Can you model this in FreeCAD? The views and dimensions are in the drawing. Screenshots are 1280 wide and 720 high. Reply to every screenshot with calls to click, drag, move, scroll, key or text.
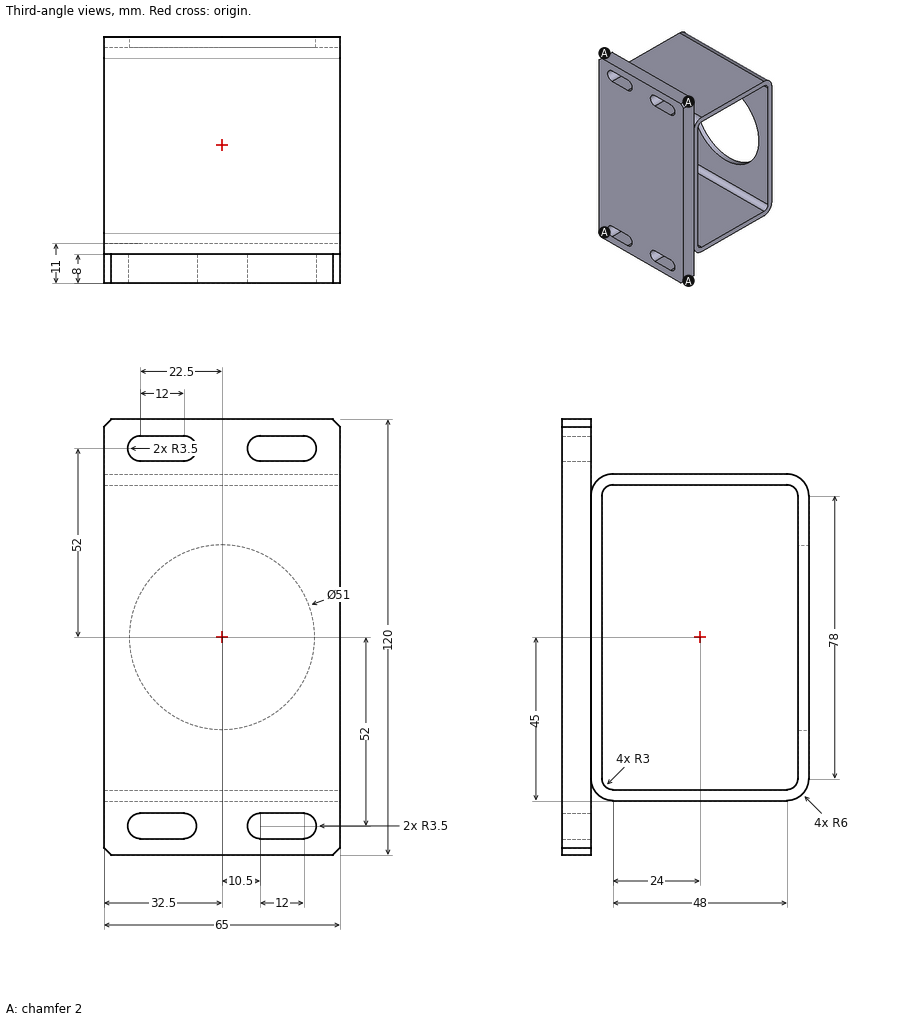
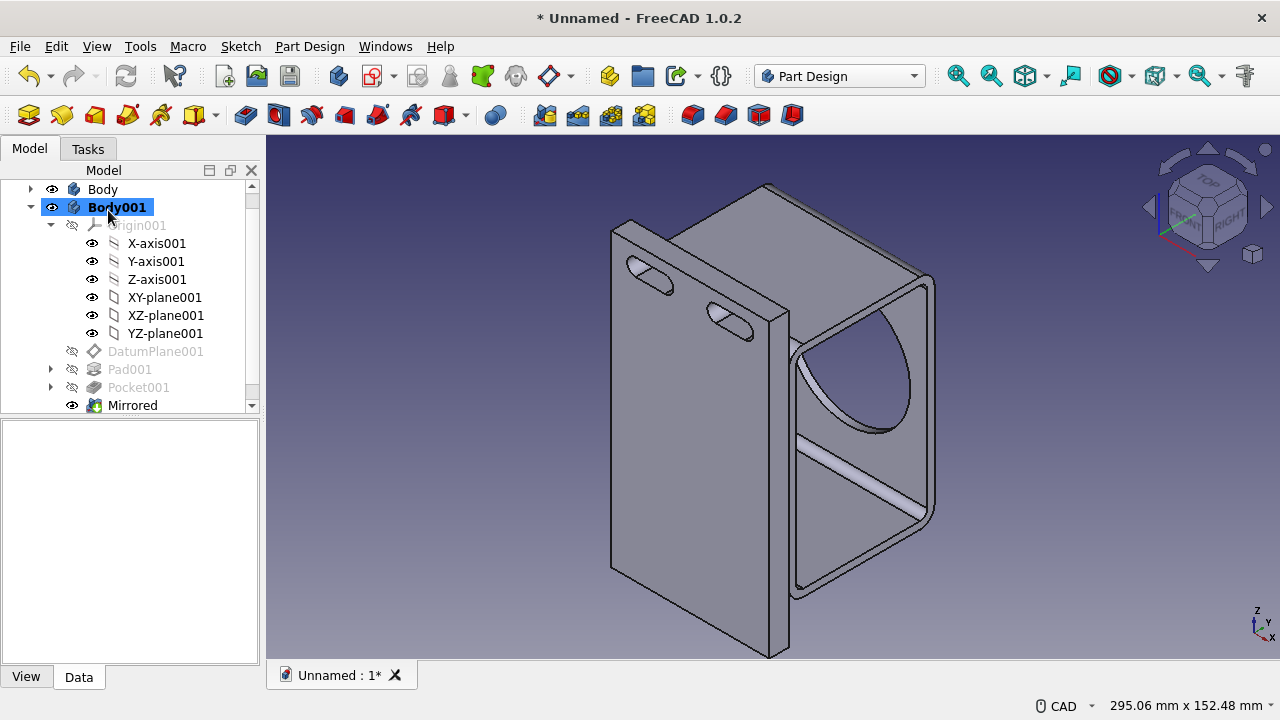
click(117, 387)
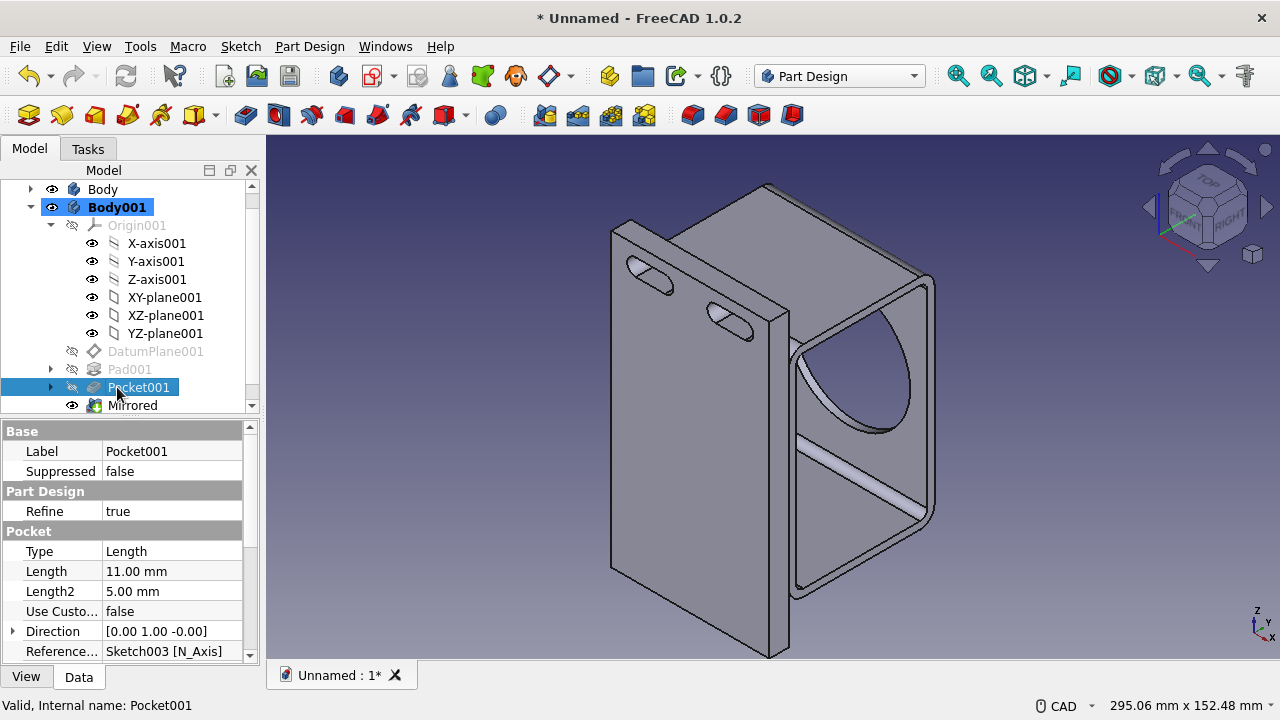
click(545, 116)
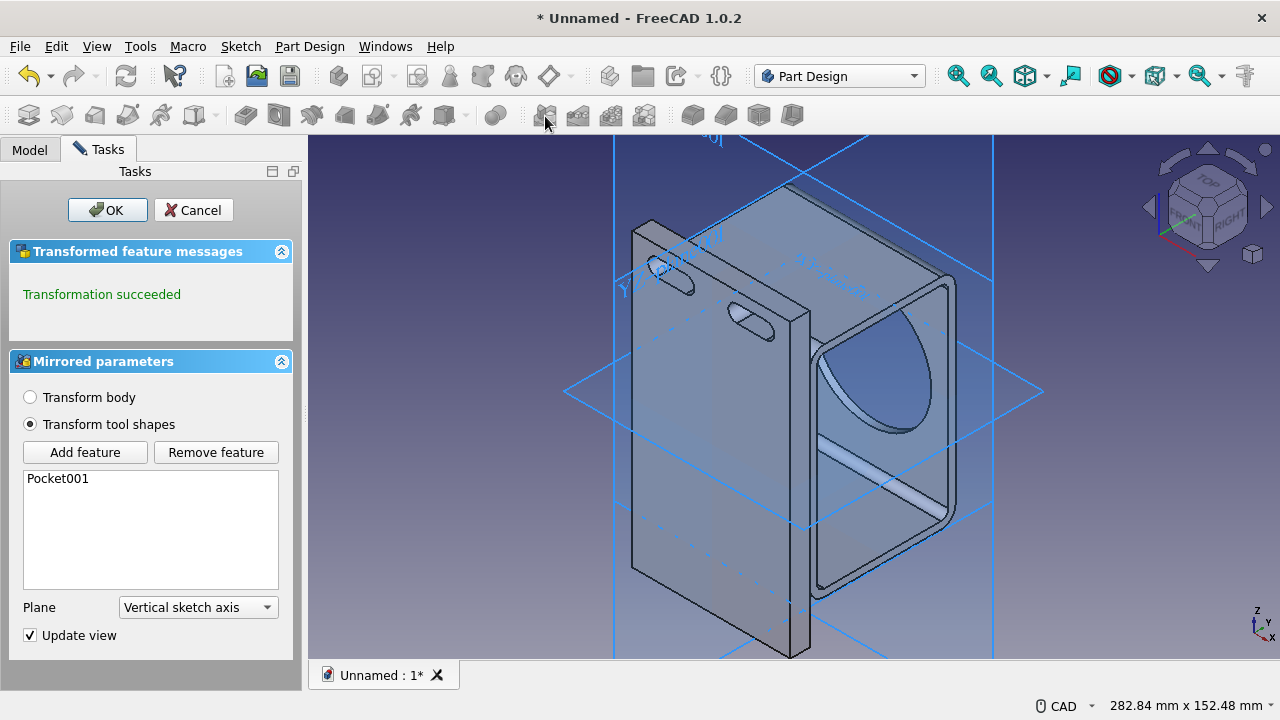
click(199, 608)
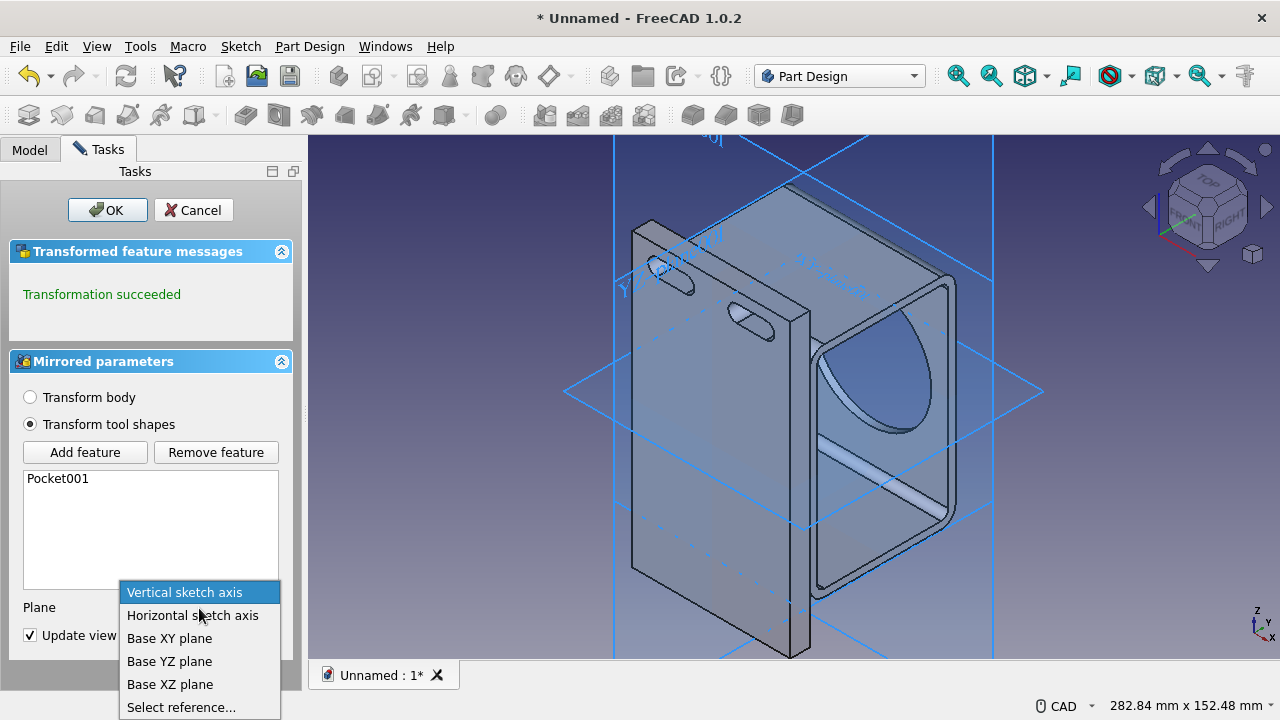
click(198, 638)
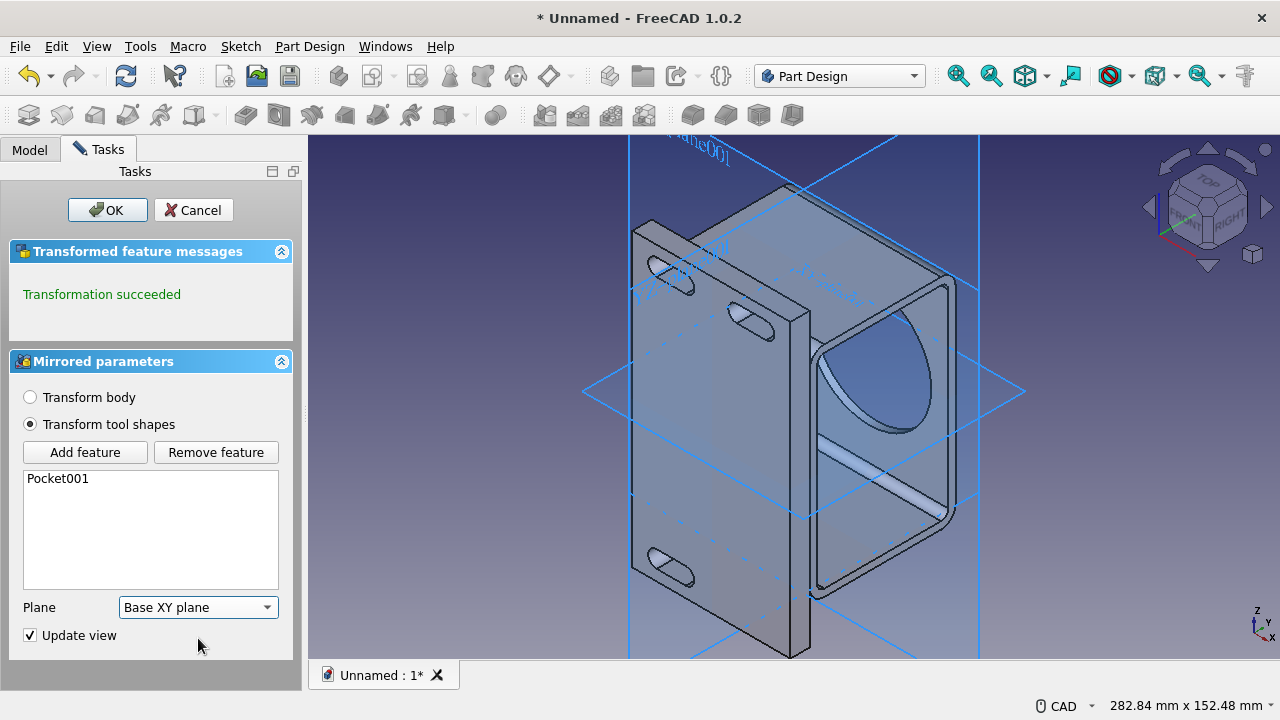
click(108, 210)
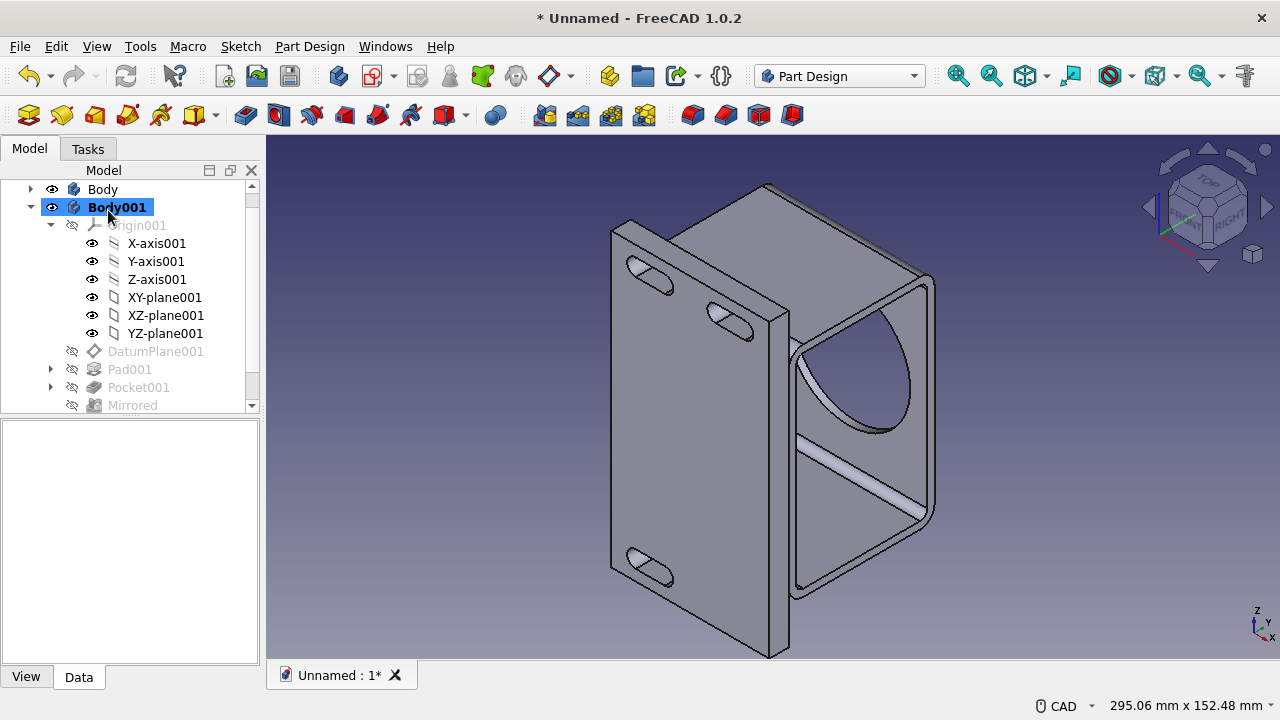
click(690, 396)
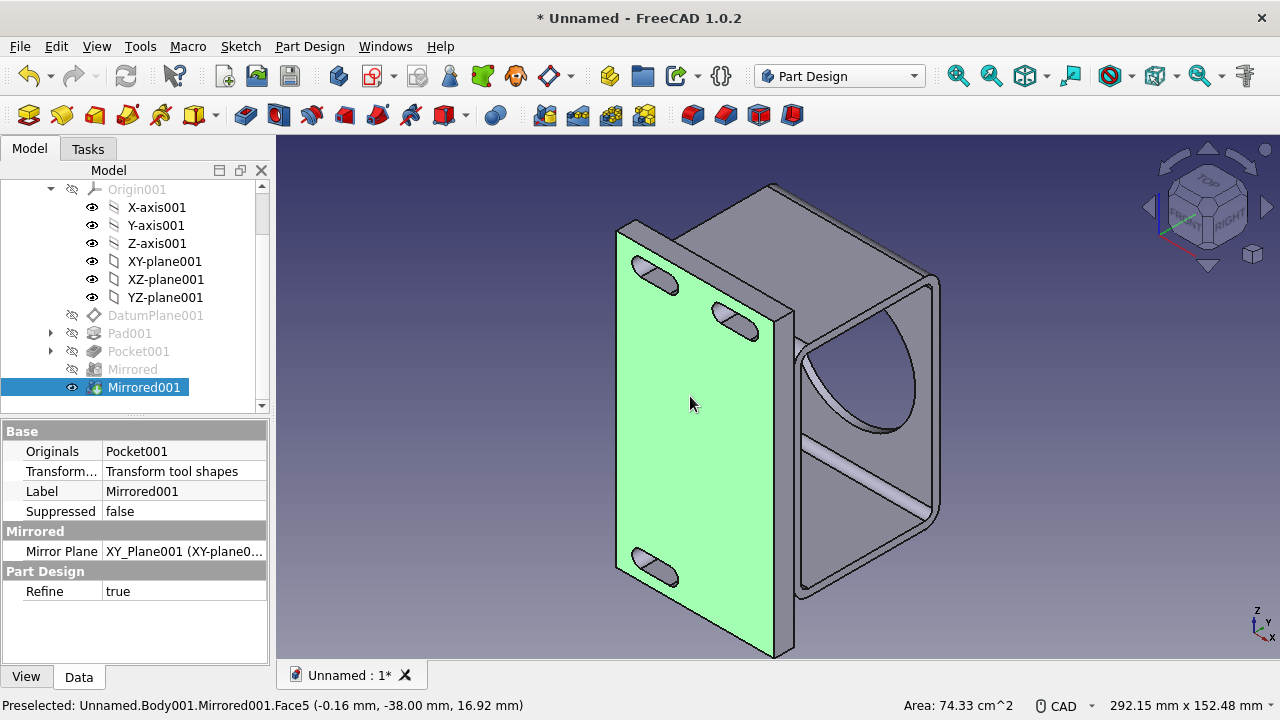
click(372, 76)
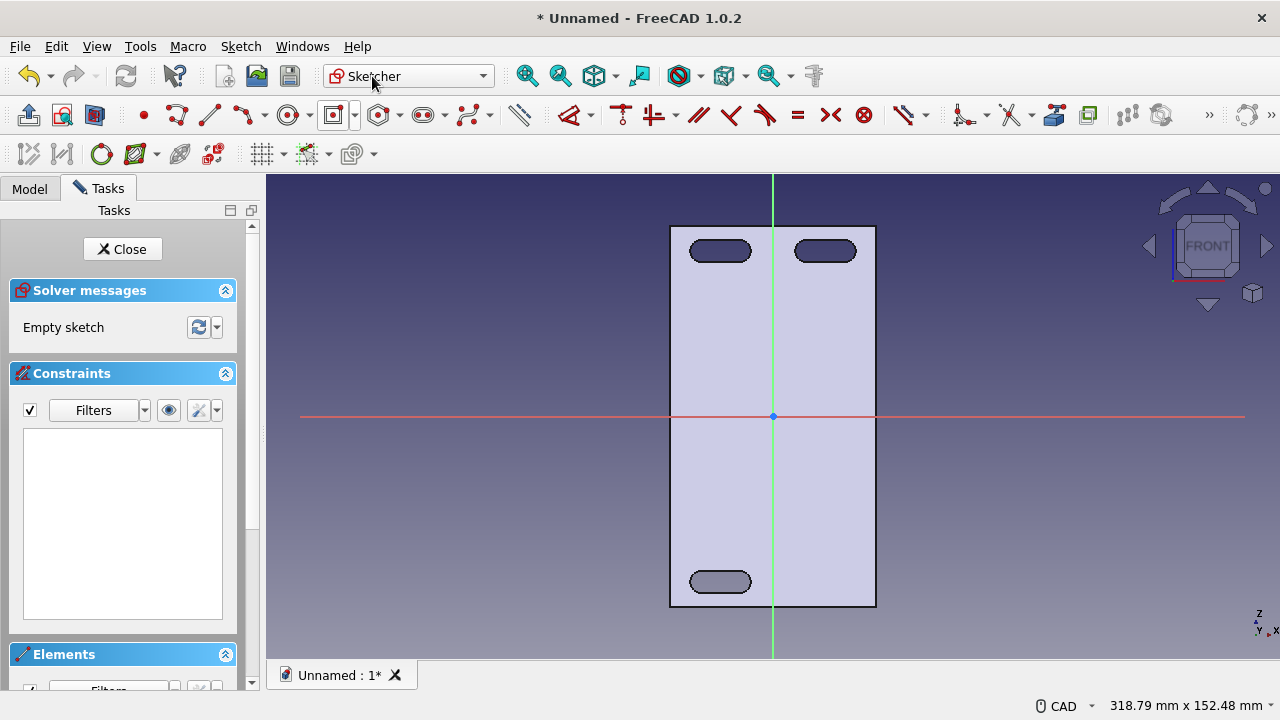
scroll(841, 603, up, 11)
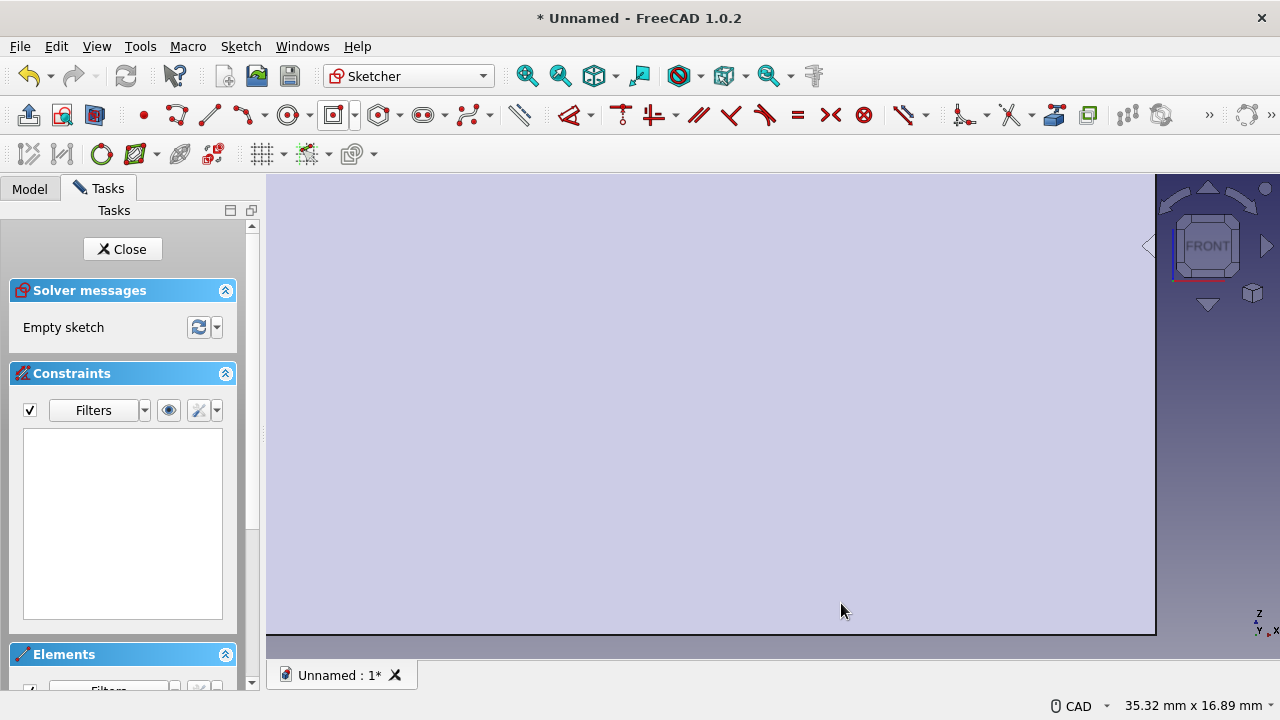
click(422, 116)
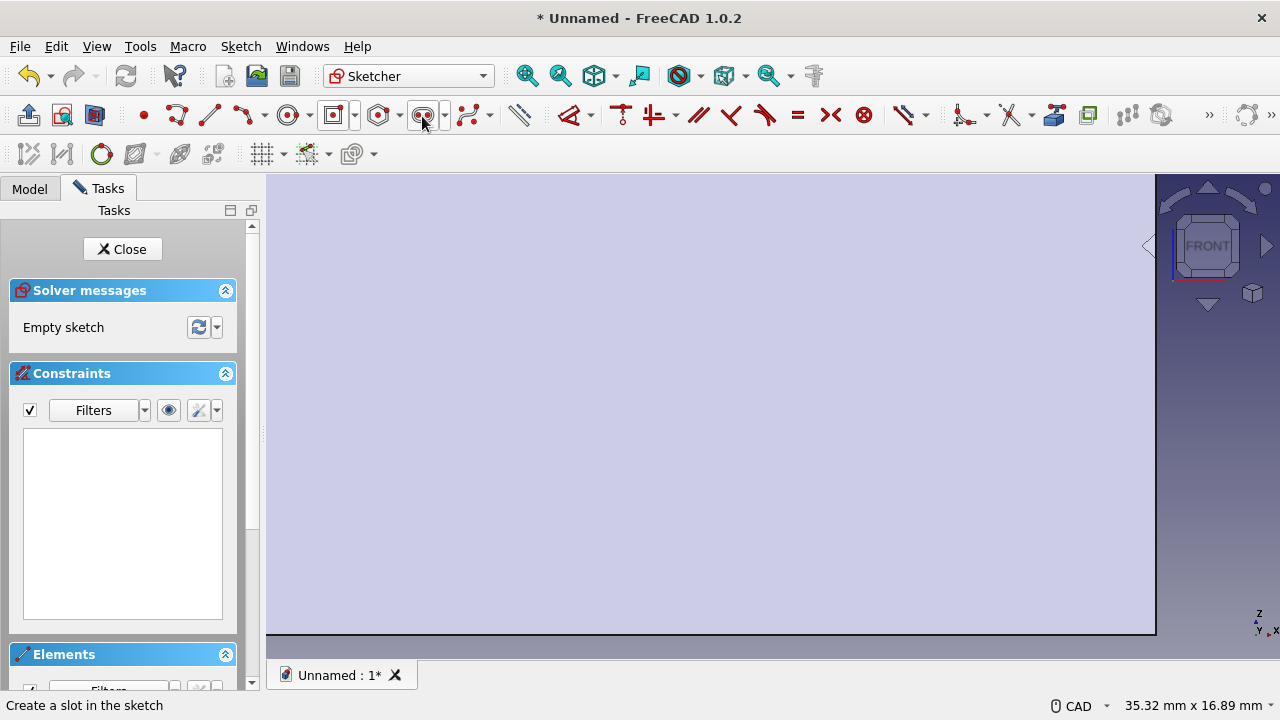
click(524, 405)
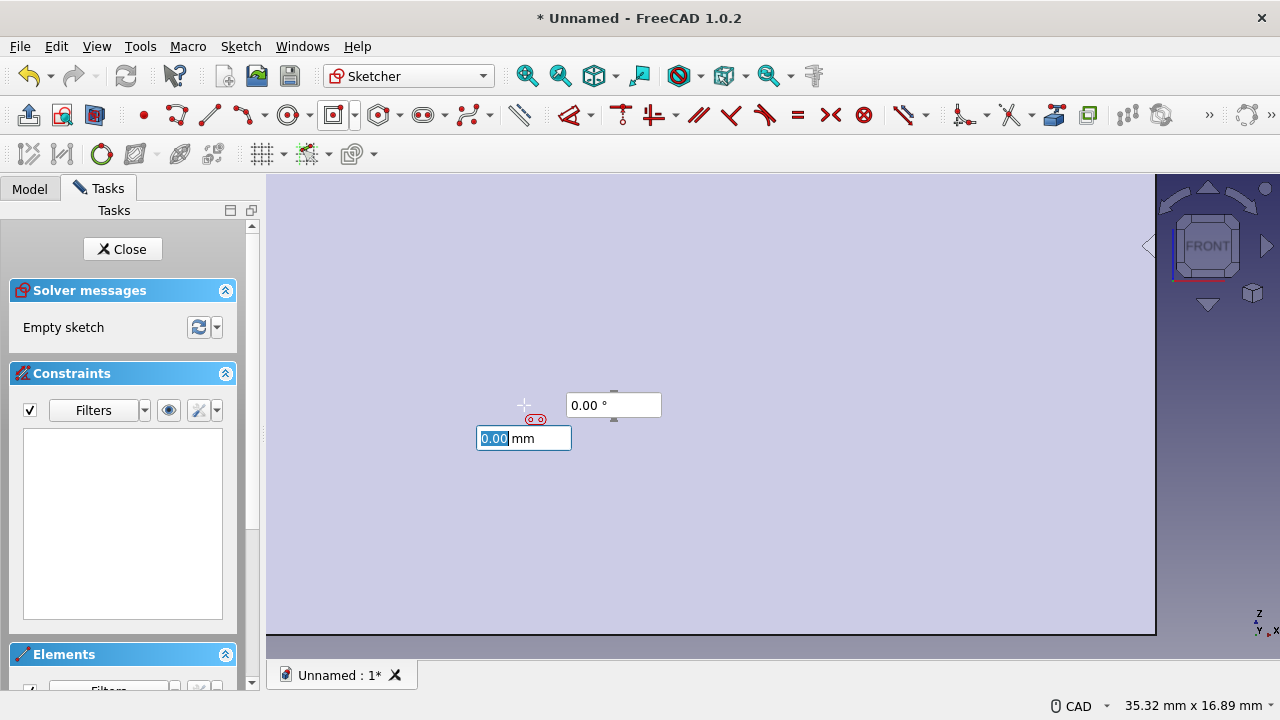
click(869, 405)